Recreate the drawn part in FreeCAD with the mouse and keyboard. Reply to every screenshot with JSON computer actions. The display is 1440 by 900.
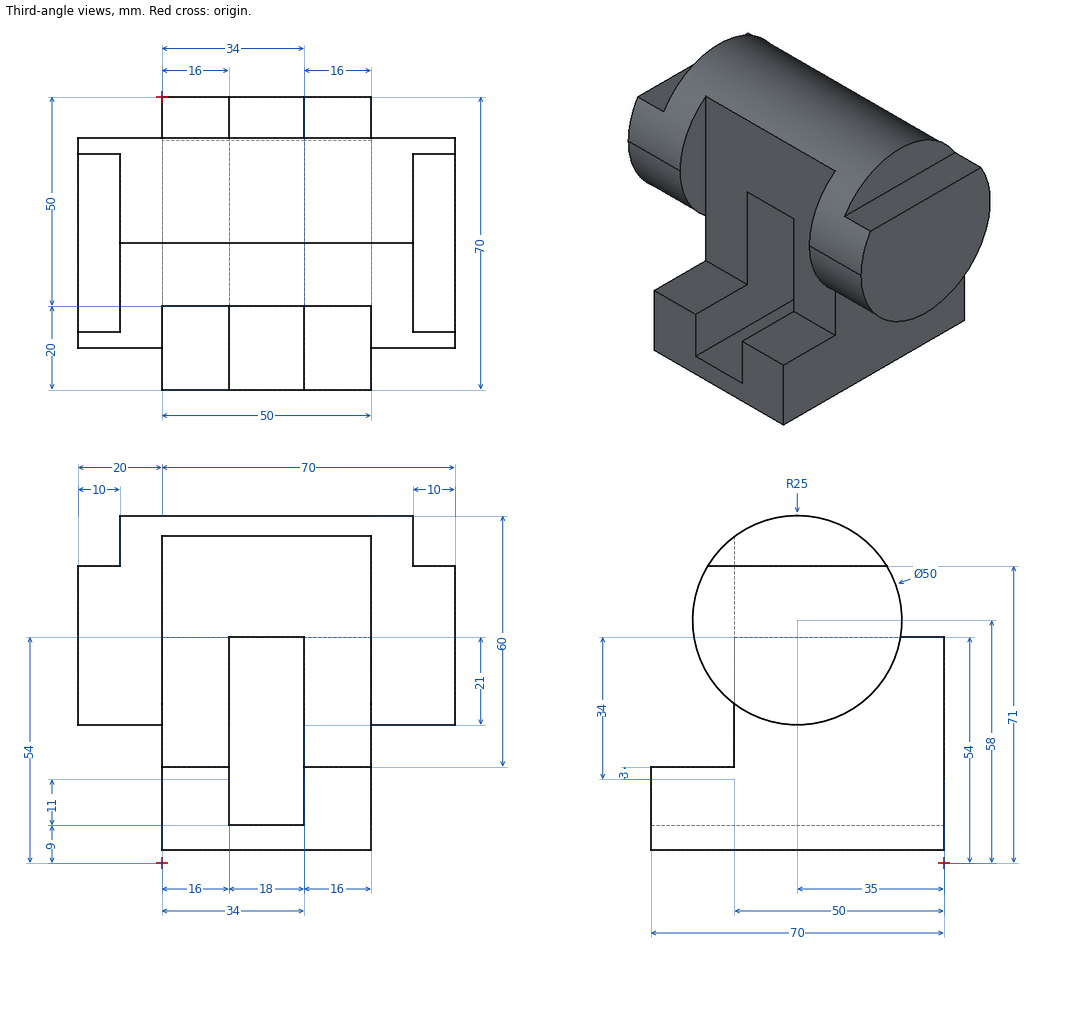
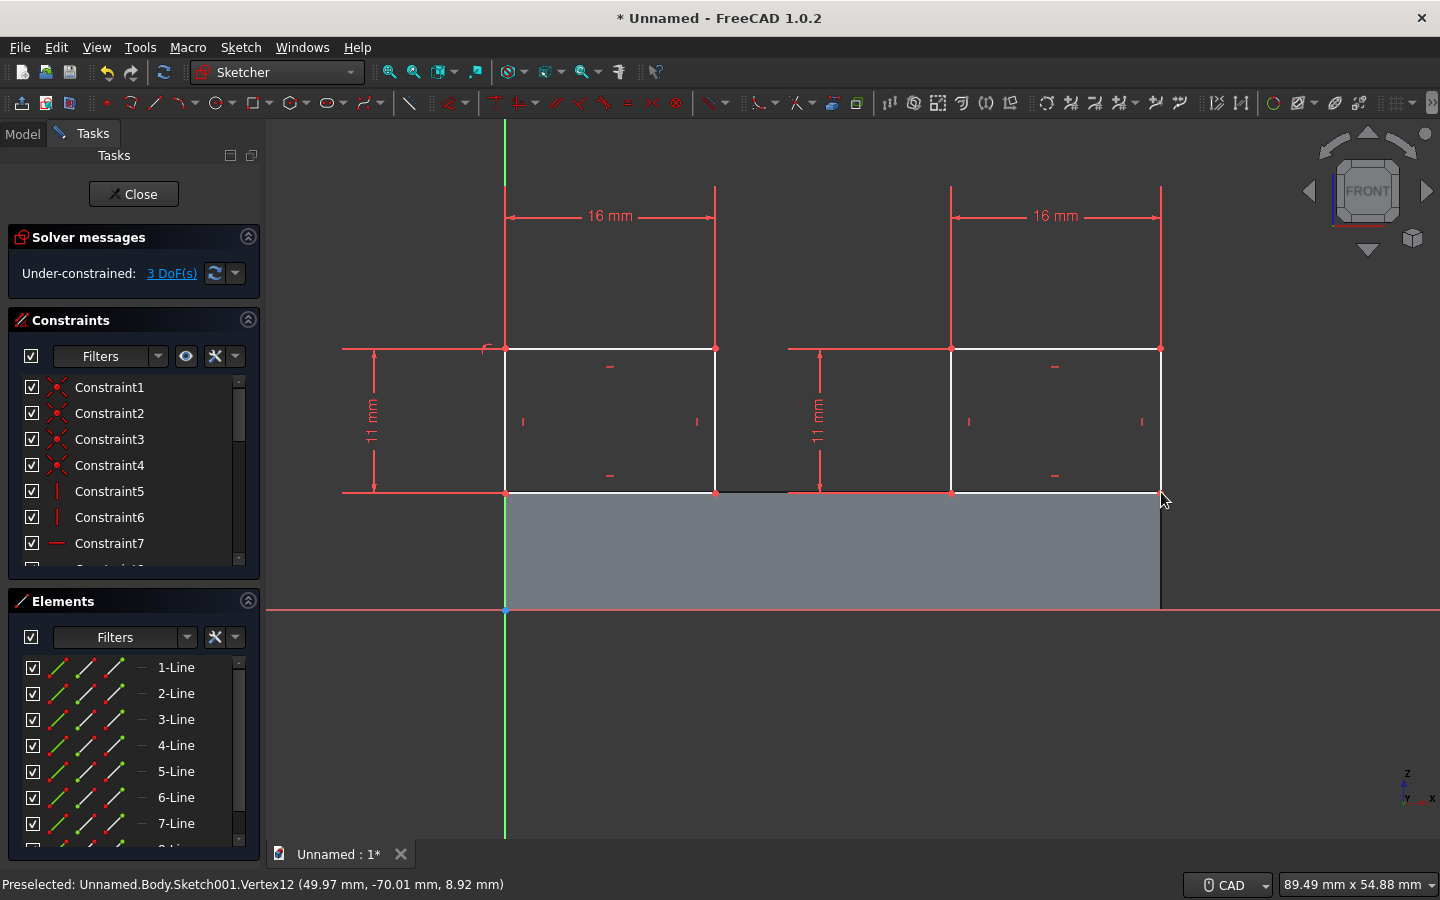
{"action": "left_click", "coordinate": [505, 493]}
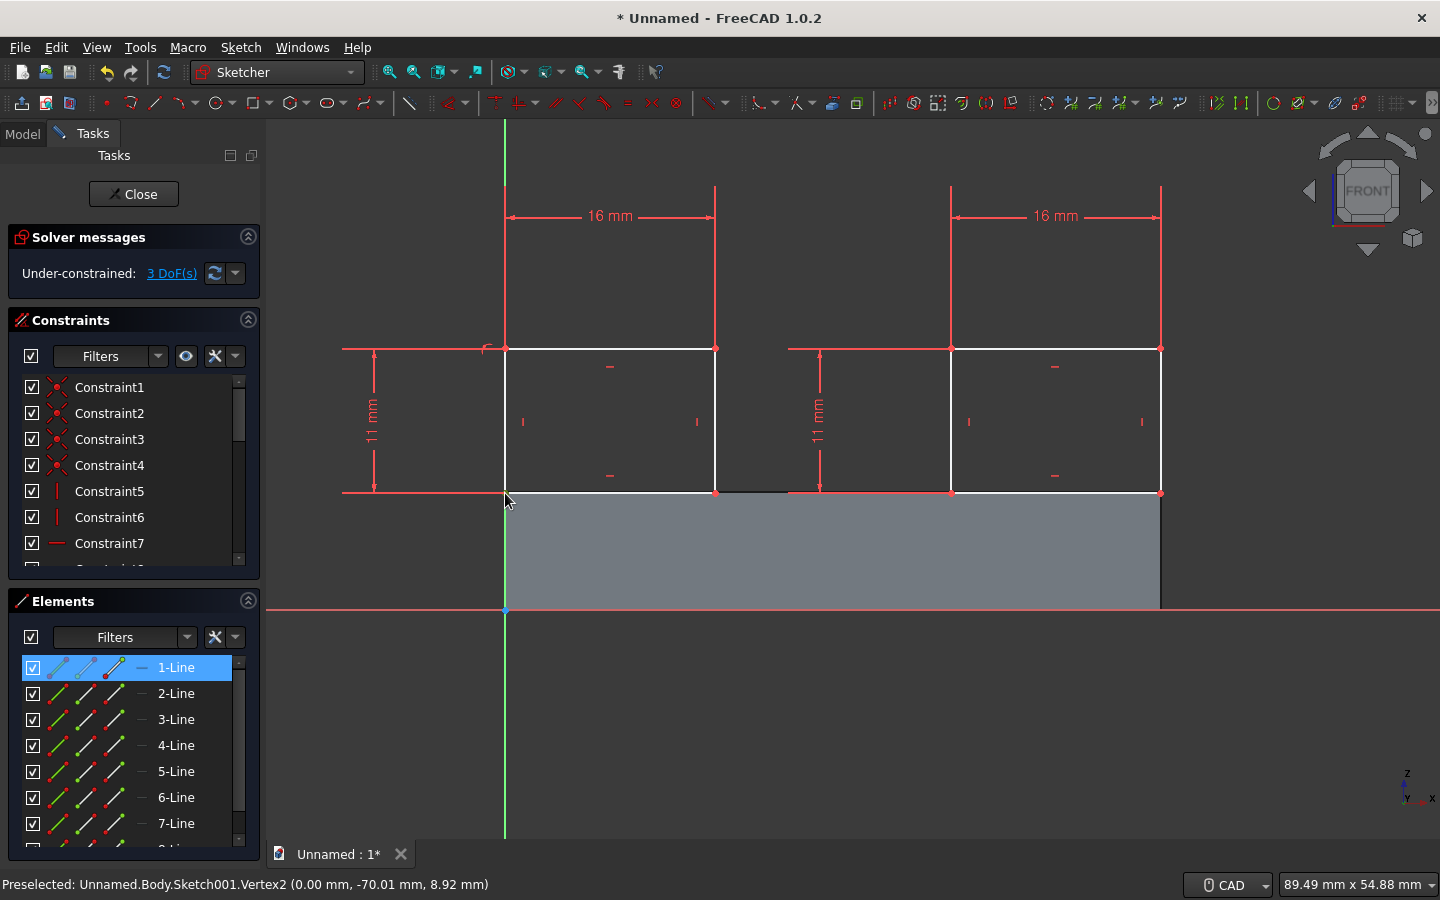
{"action": "key", "text": "i"}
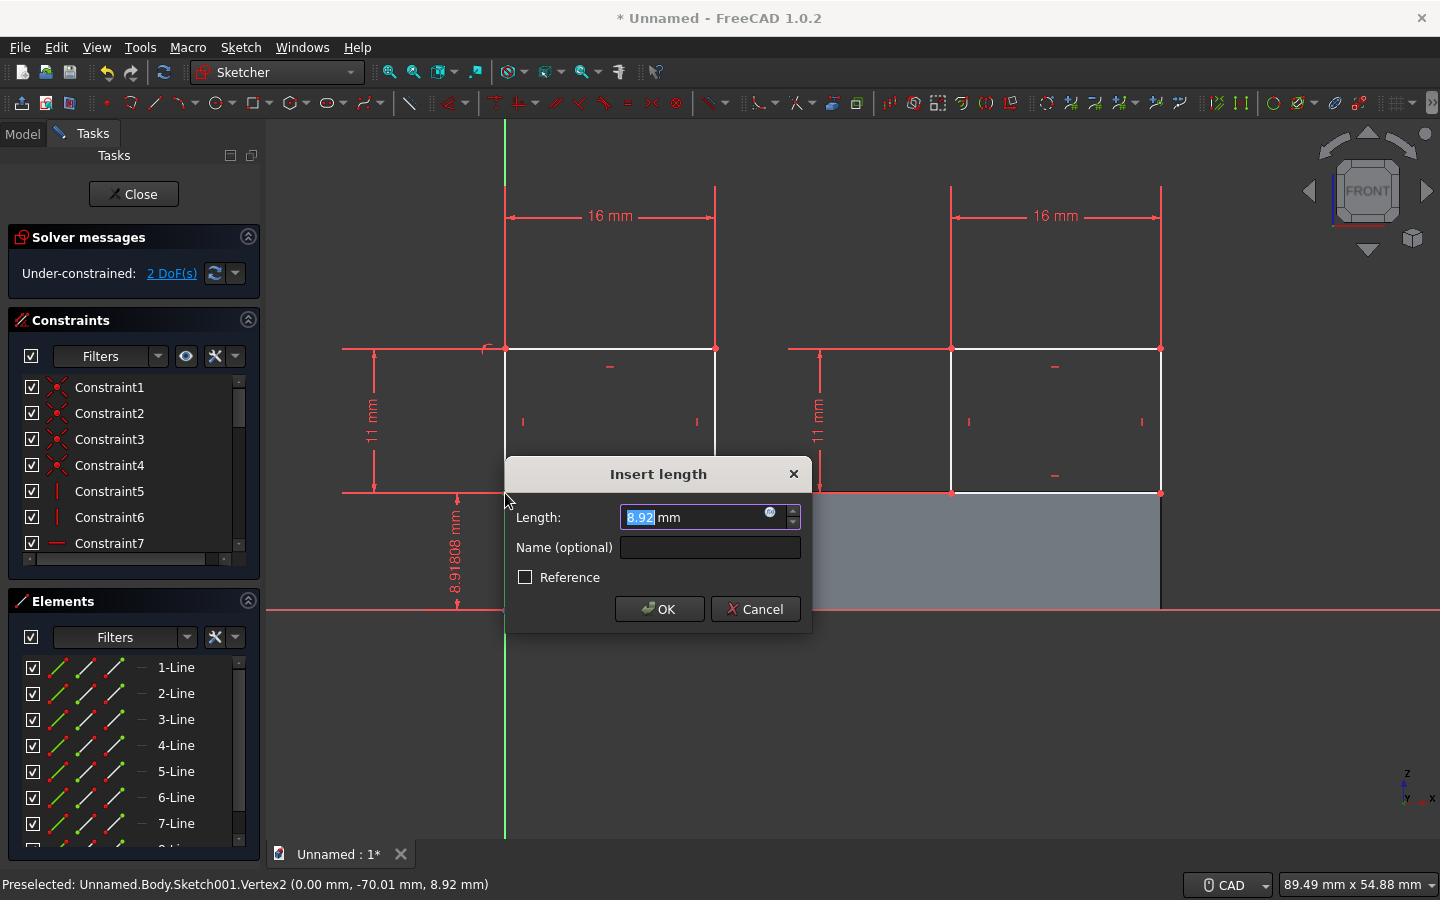
{"action": "type", "text": "9"}
{"action": "key", "text": "Return"}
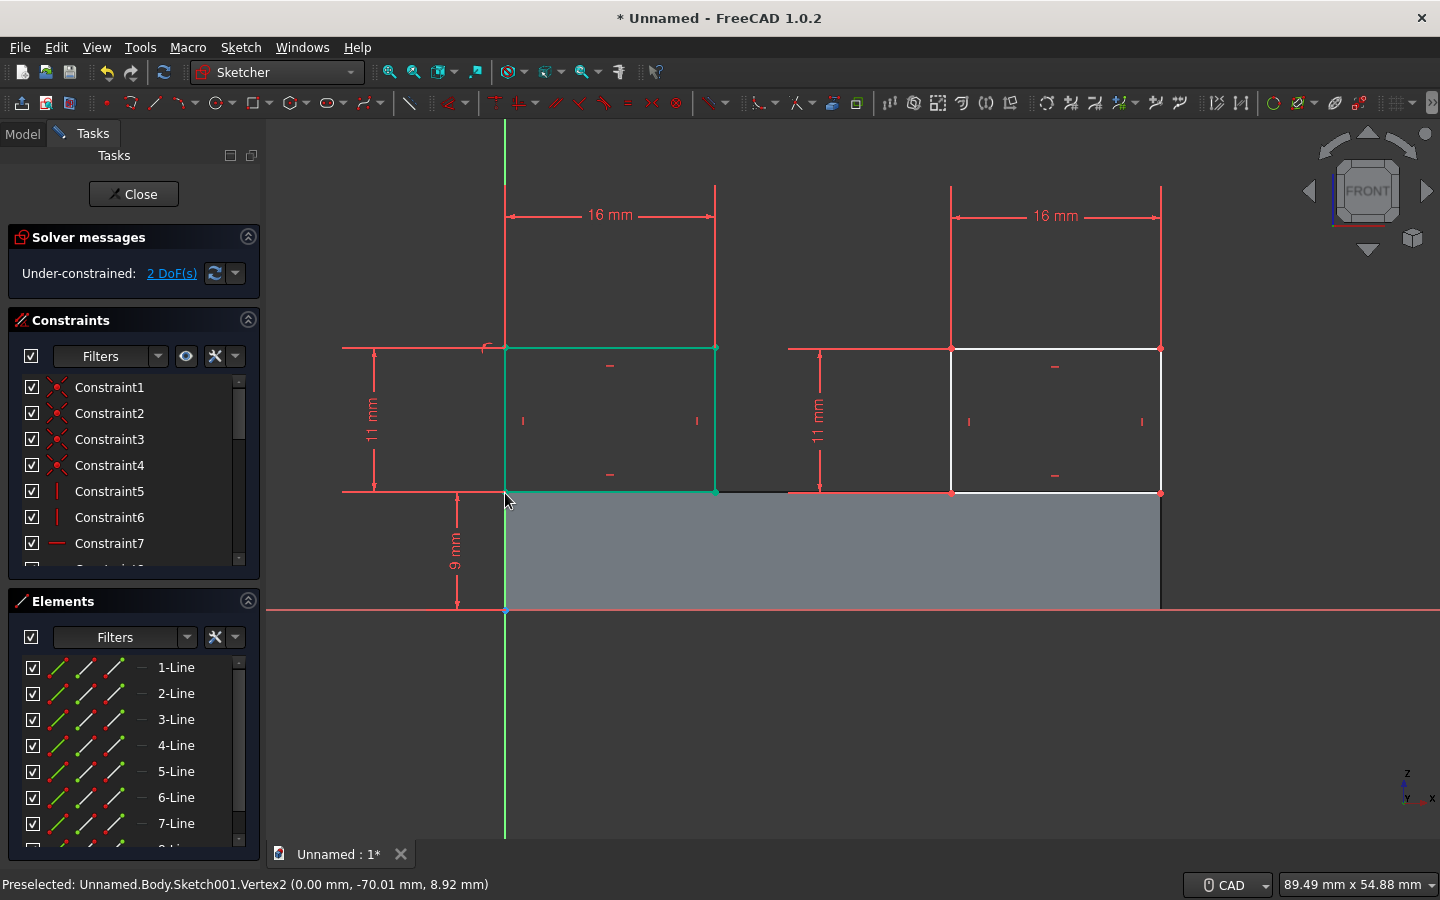
{"action": "left_click", "coordinate": [951, 493]}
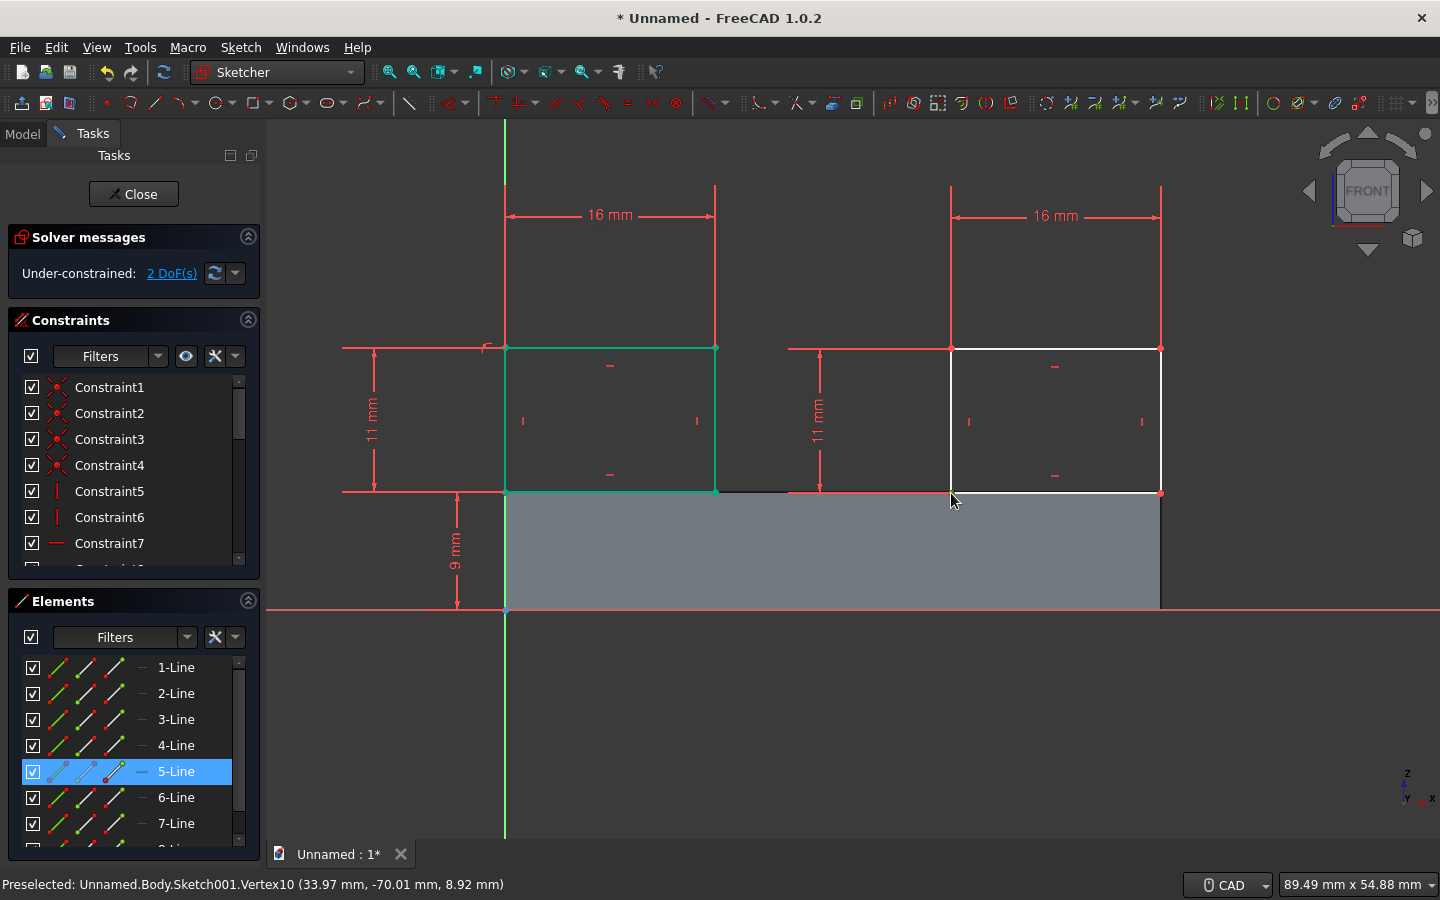
{"action": "key", "text": "i"}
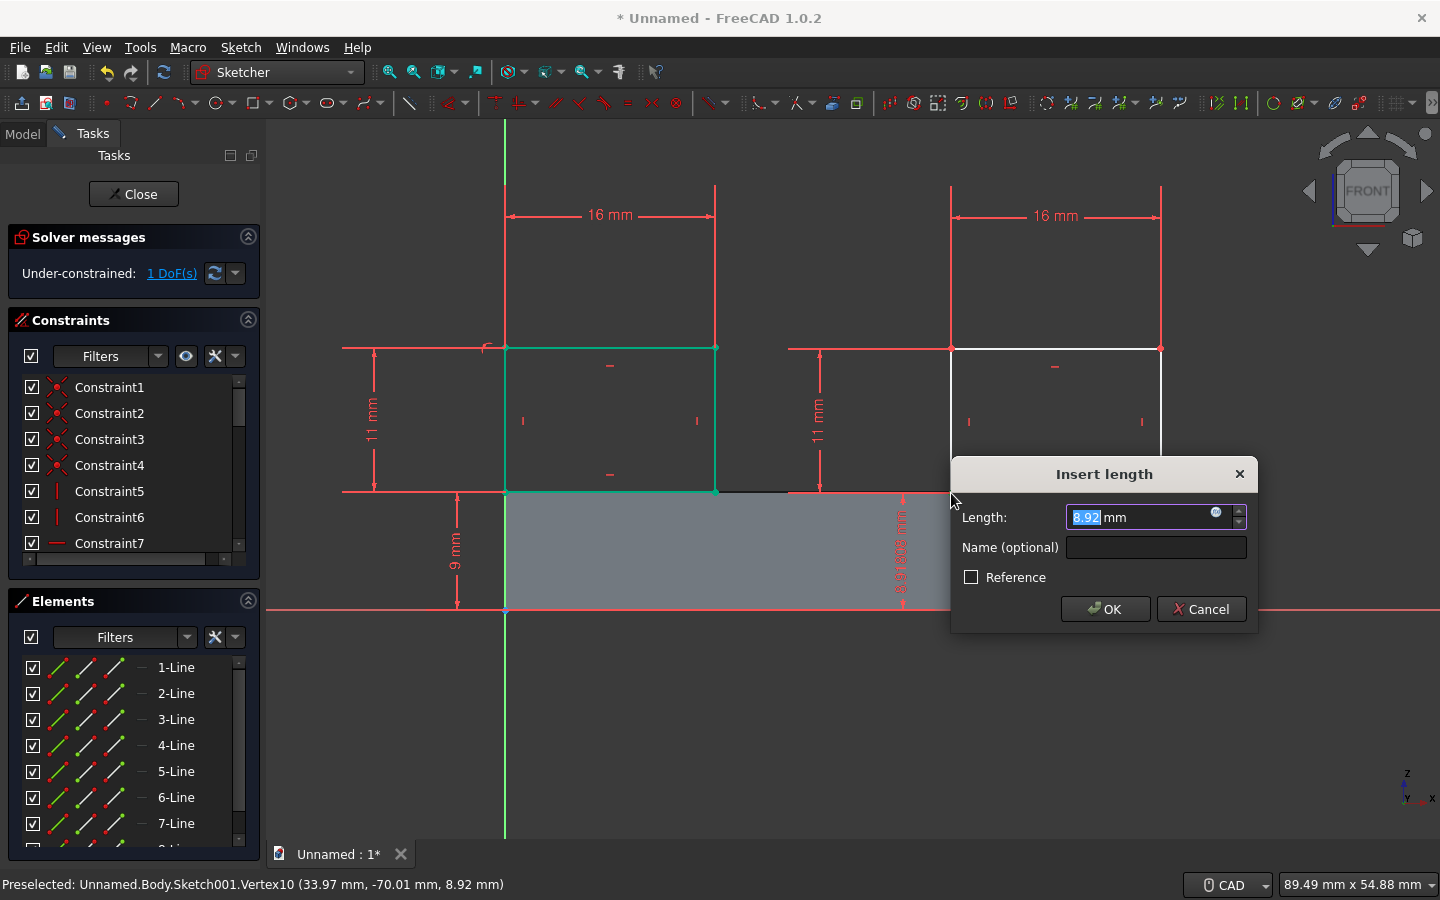
{"action": "type", "text": "9"}
{"action": "key", "text": "Return"}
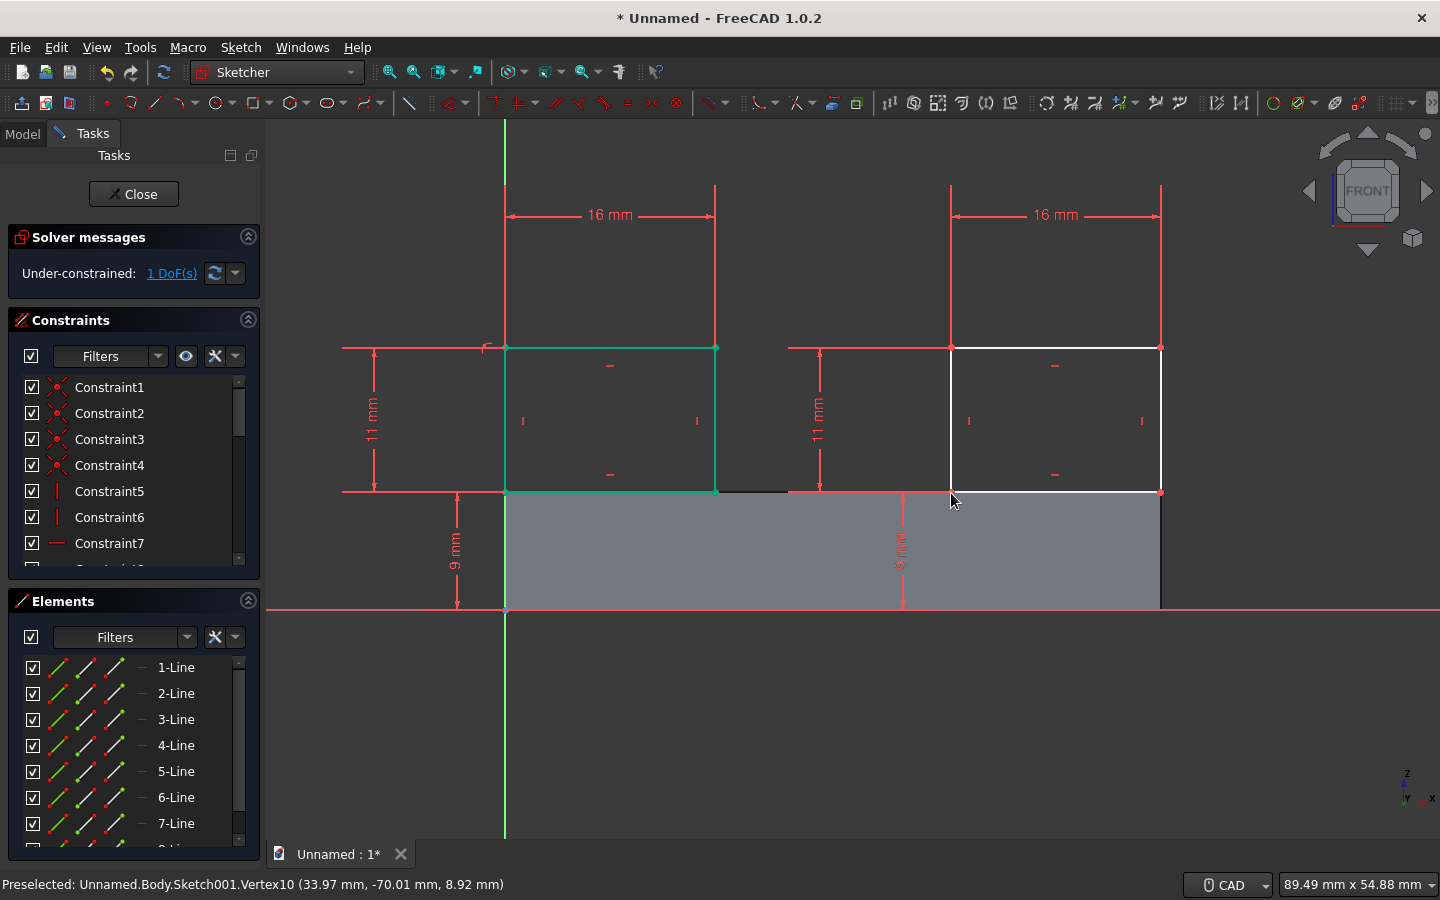
{"action": "left_click", "coordinate": [951, 348]}